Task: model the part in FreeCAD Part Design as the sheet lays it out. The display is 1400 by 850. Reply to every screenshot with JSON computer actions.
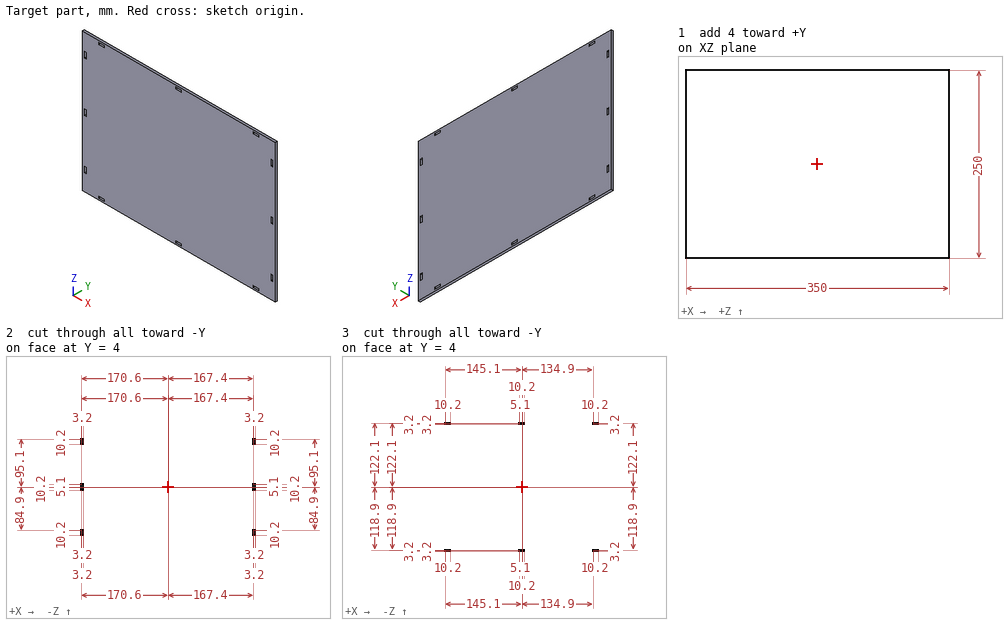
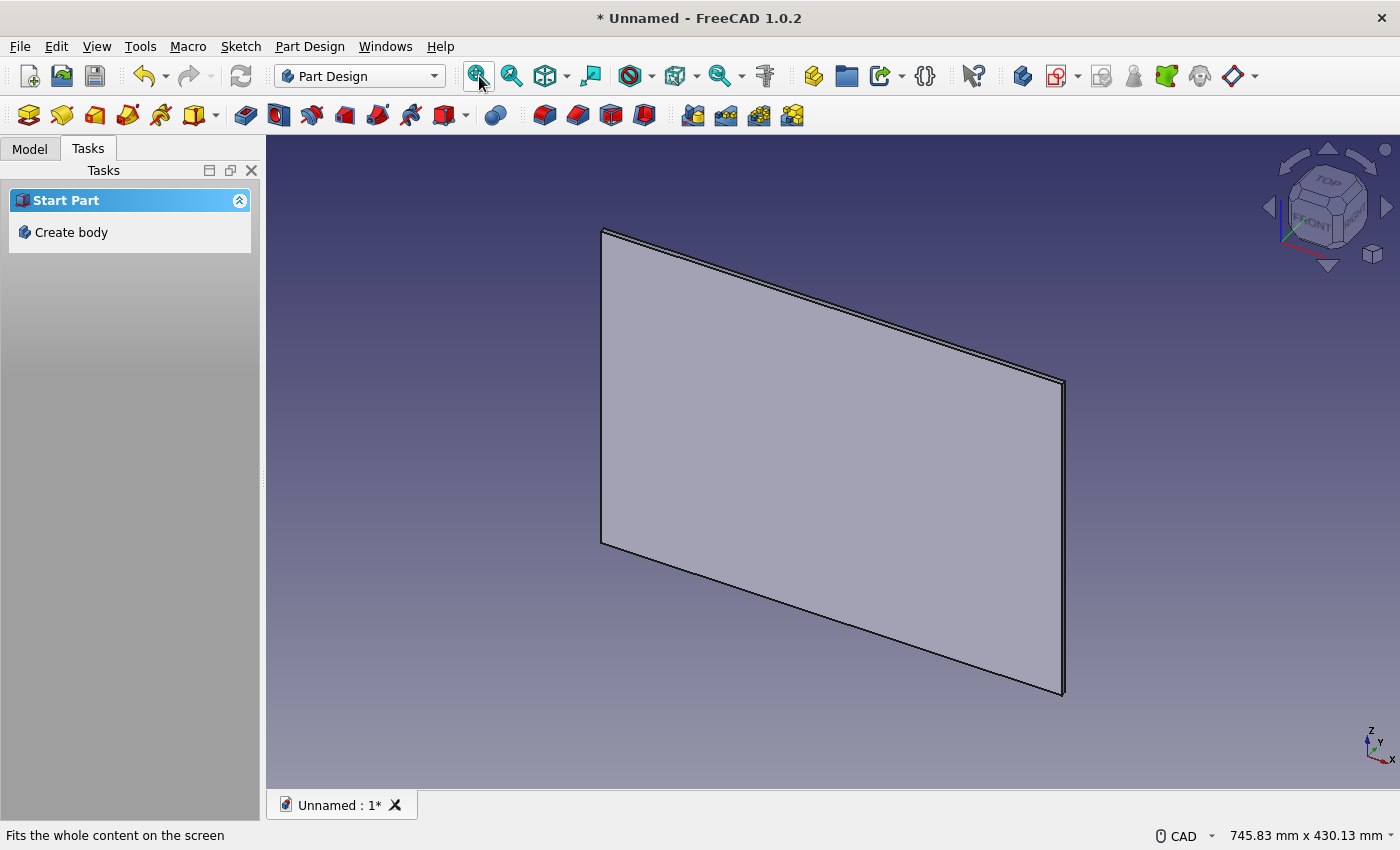
{"action": "key", "text": "4"}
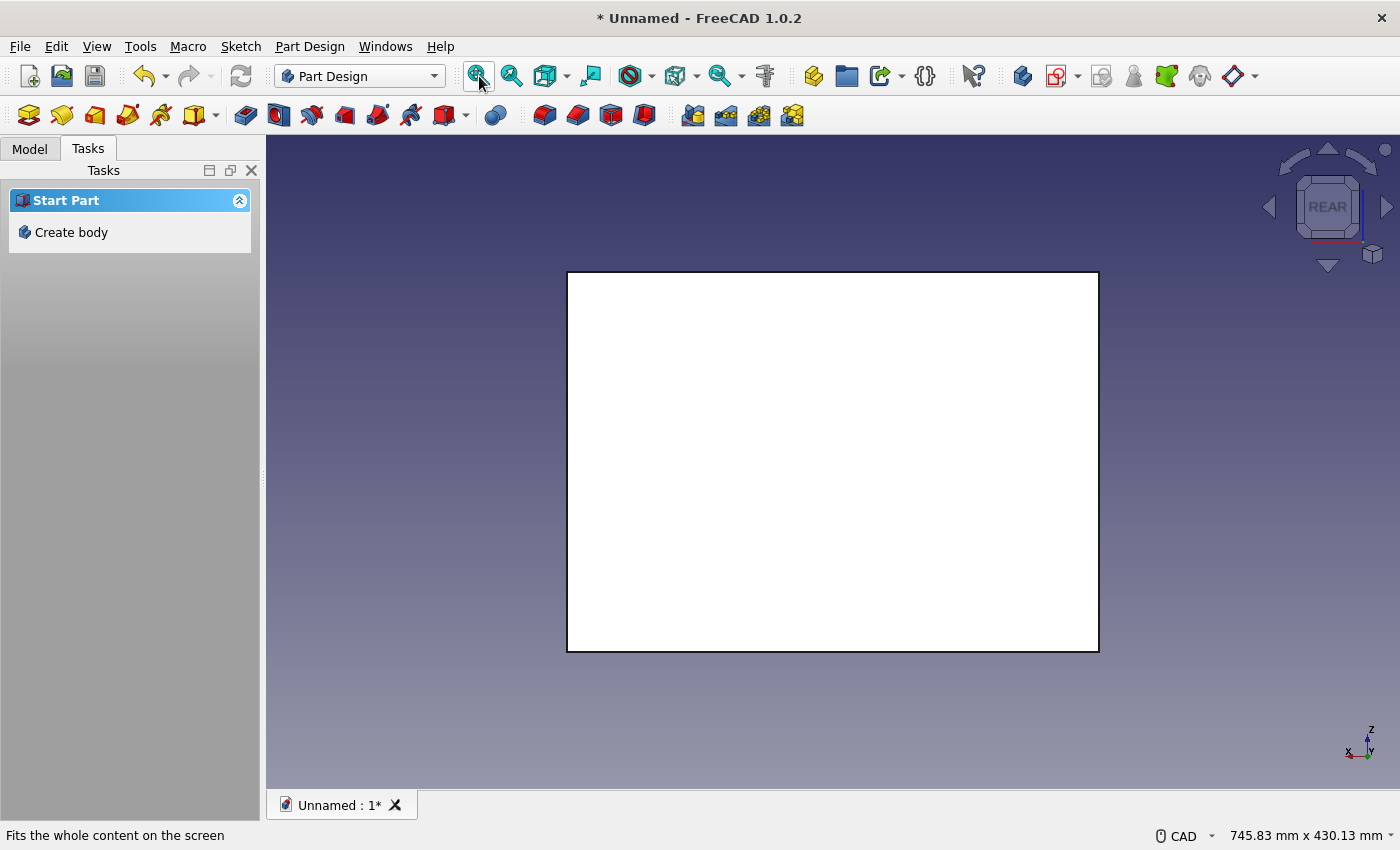
{"action": "left_click", "coordinate": [833, 461]}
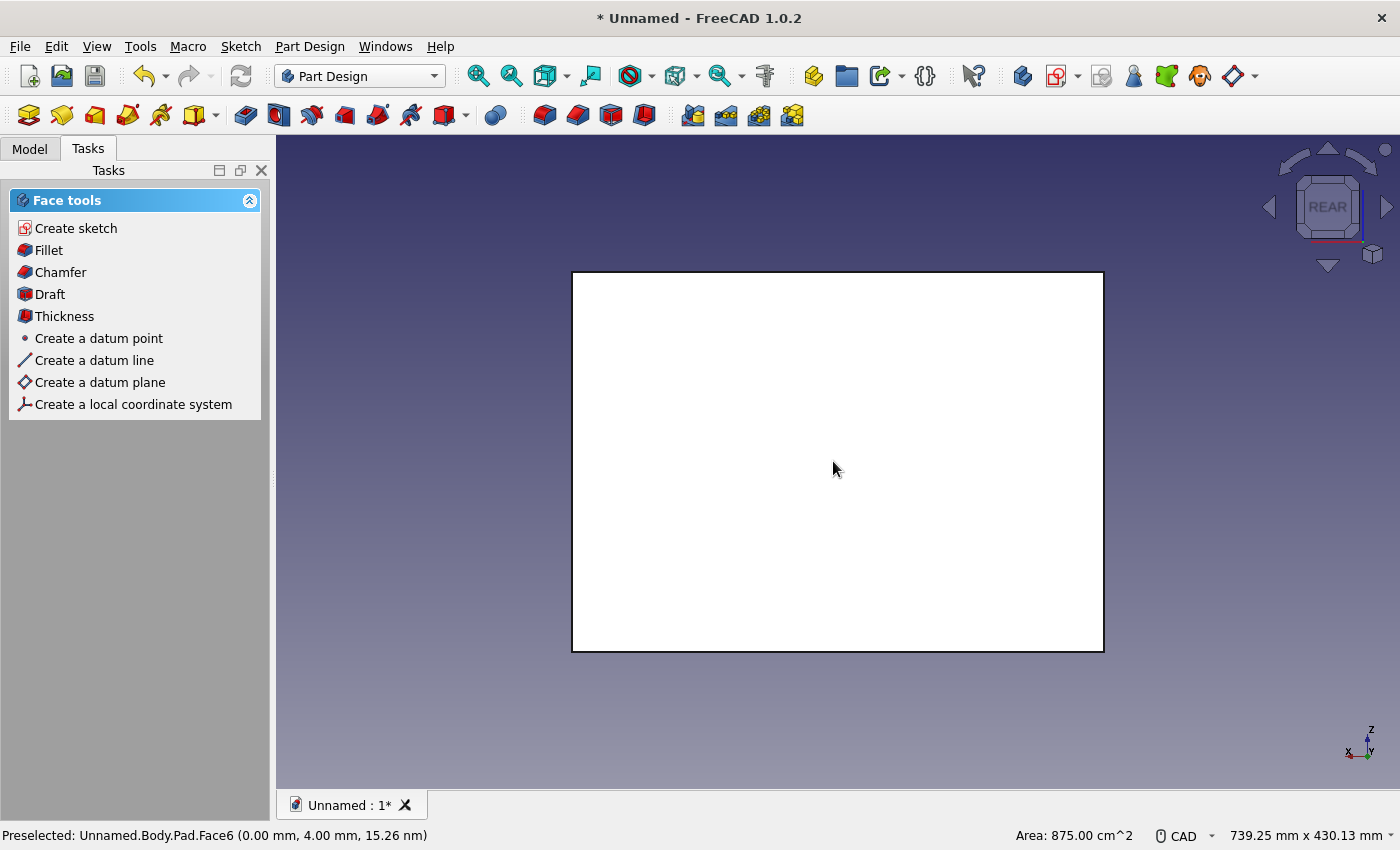
{"action": "left_click", "coordinate": [1056, 76]}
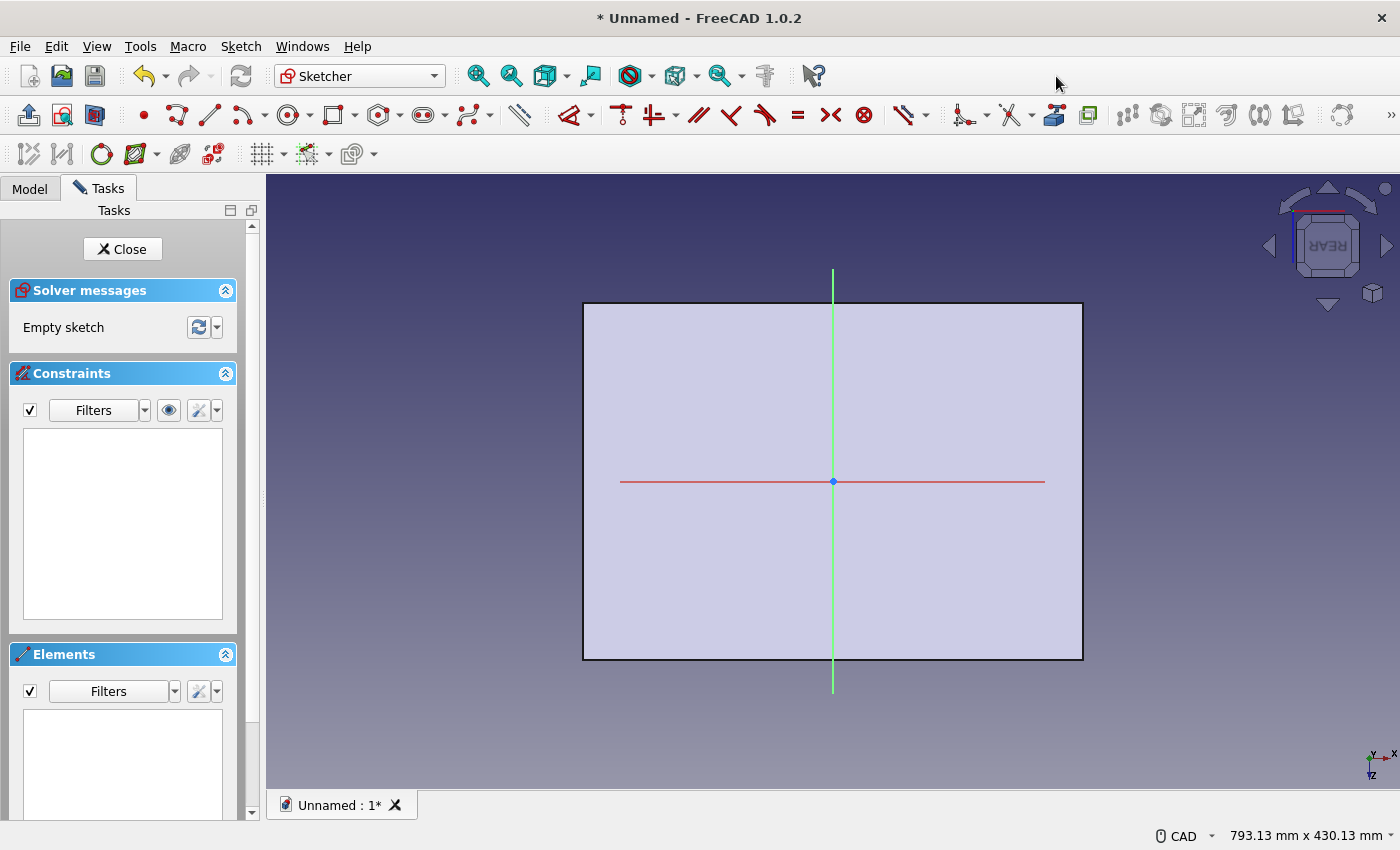
{"action": "scroll", "coordinate": [972, 481], "scroll_direction": "up", "scroll_amount": 2}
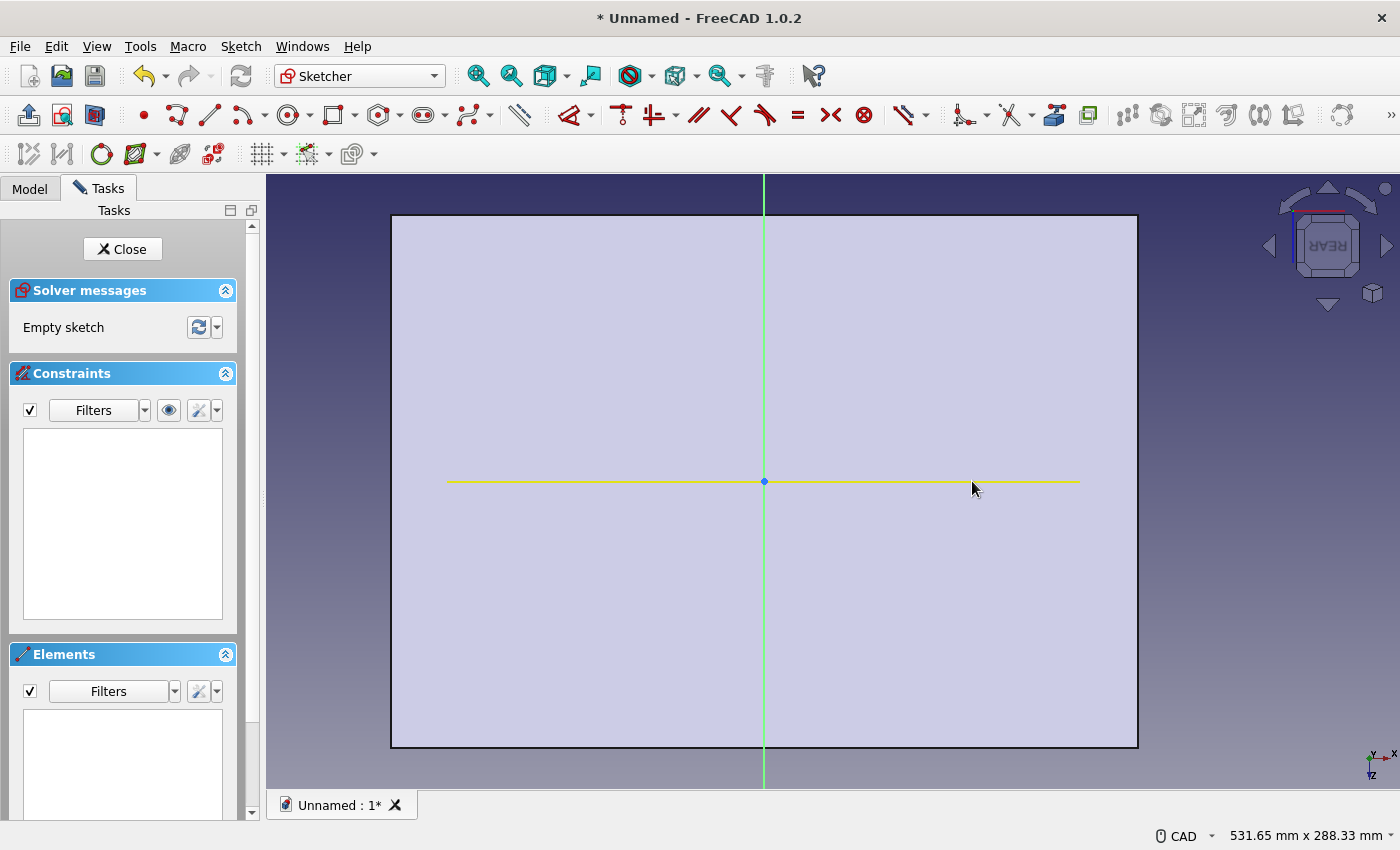
{"action": "left_click", "coordinate": [332, 116]}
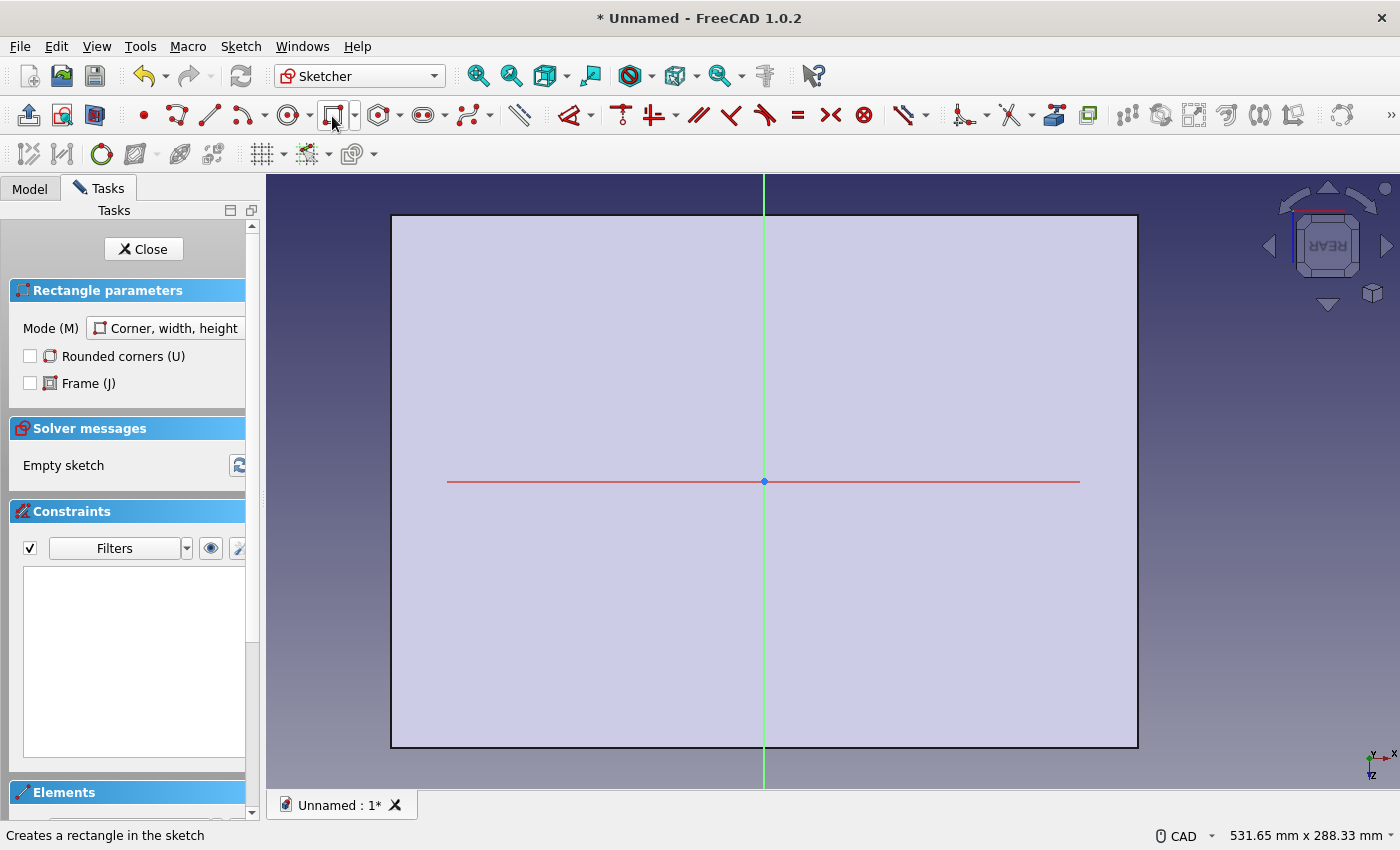
{"action": "scroll", "coordinate": [400, 279], "scroll_direction": "up", "scroll_amount": 5}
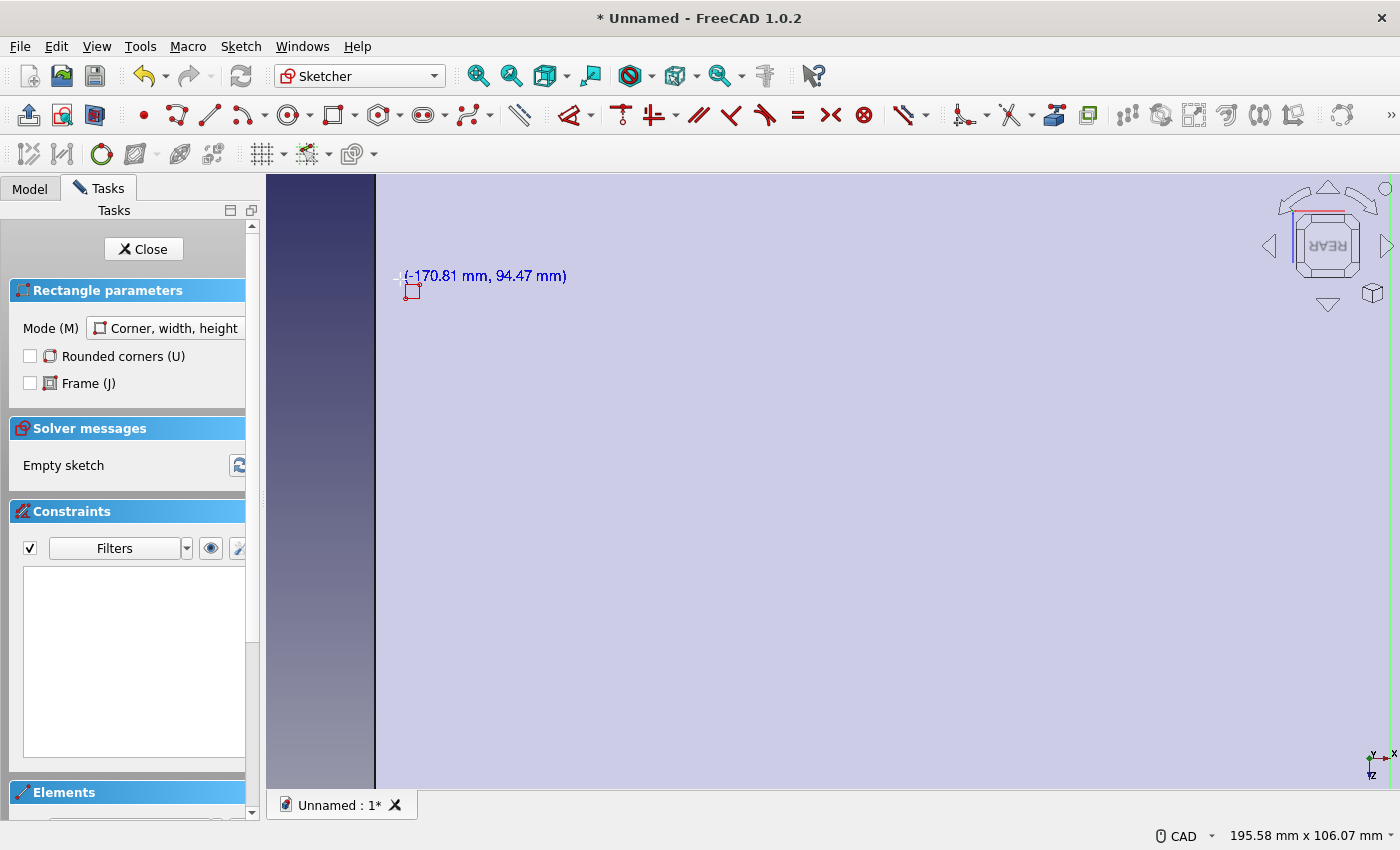
{"action": "left_click", "coordinate": [401, 278]}
{"action": "left_click", "coordinate": [420, 337]}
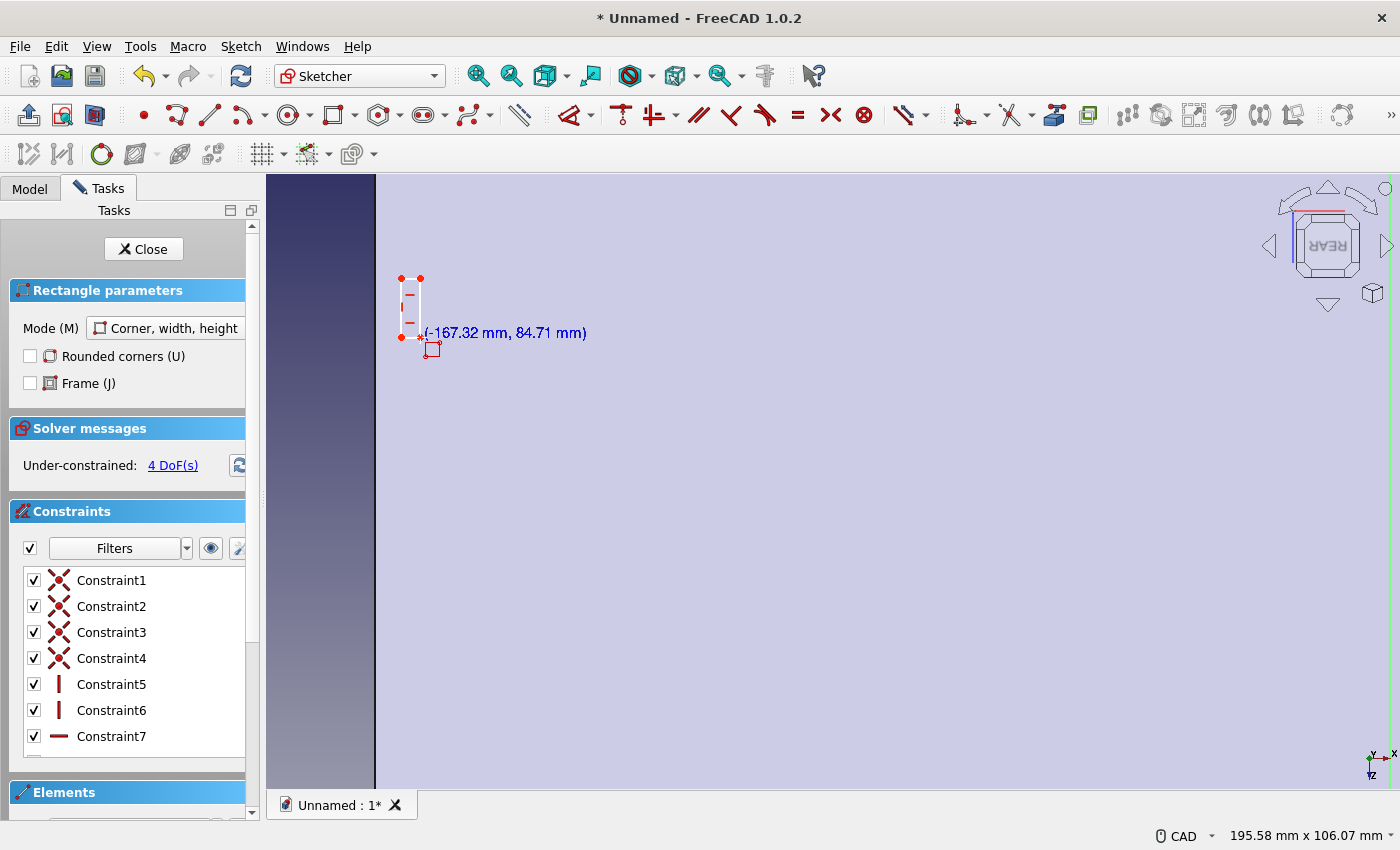
{"action": "scroll", "coordinate": [400, 279], "scroll_direction": "down", "scroll_amount": 5}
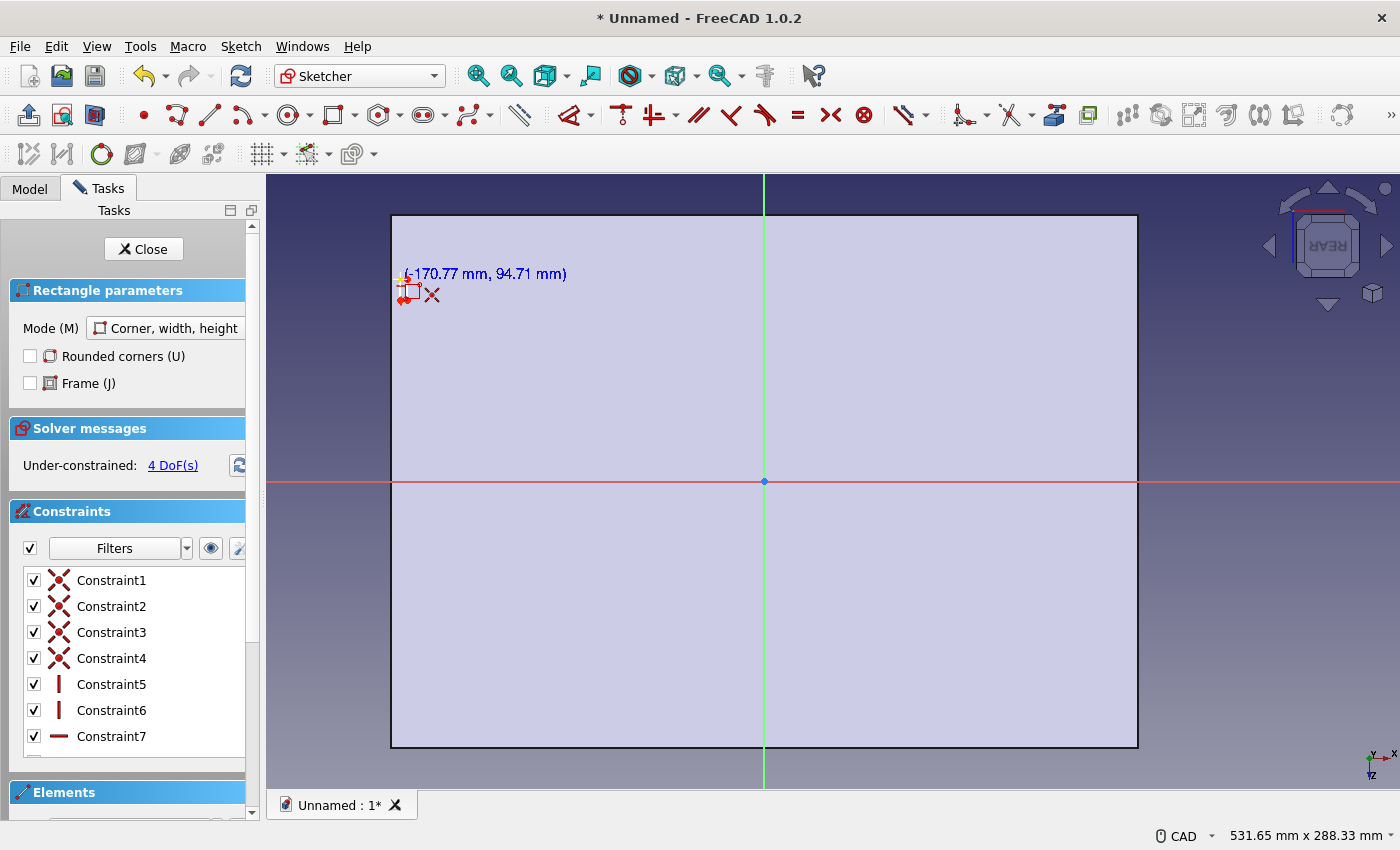
{"action": "scroll", "coordinate": [400, 471], "scroll_direction": "up", "scroll_amount": 5}